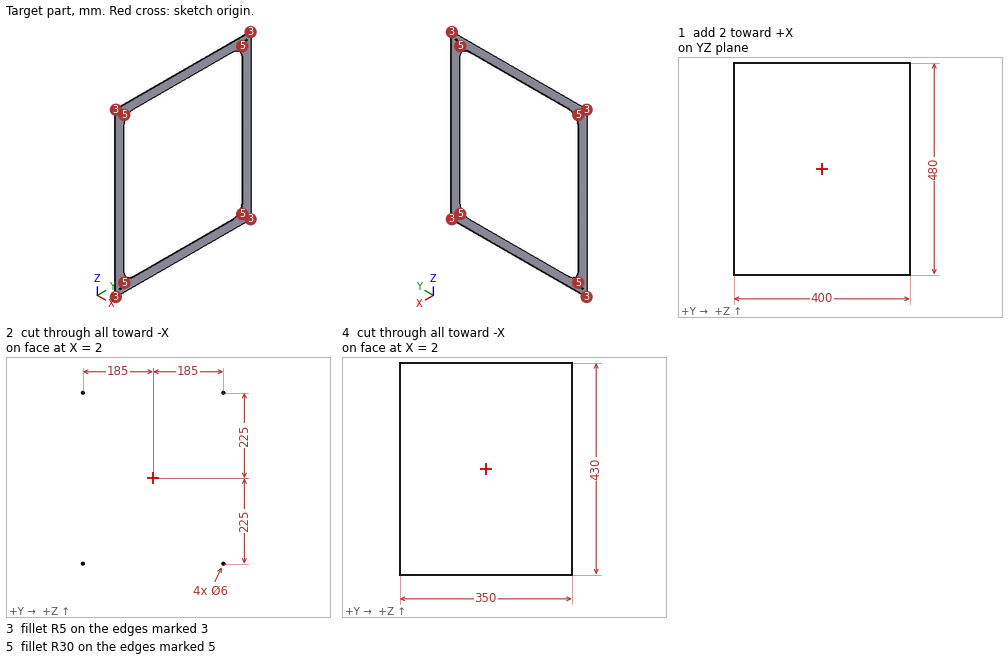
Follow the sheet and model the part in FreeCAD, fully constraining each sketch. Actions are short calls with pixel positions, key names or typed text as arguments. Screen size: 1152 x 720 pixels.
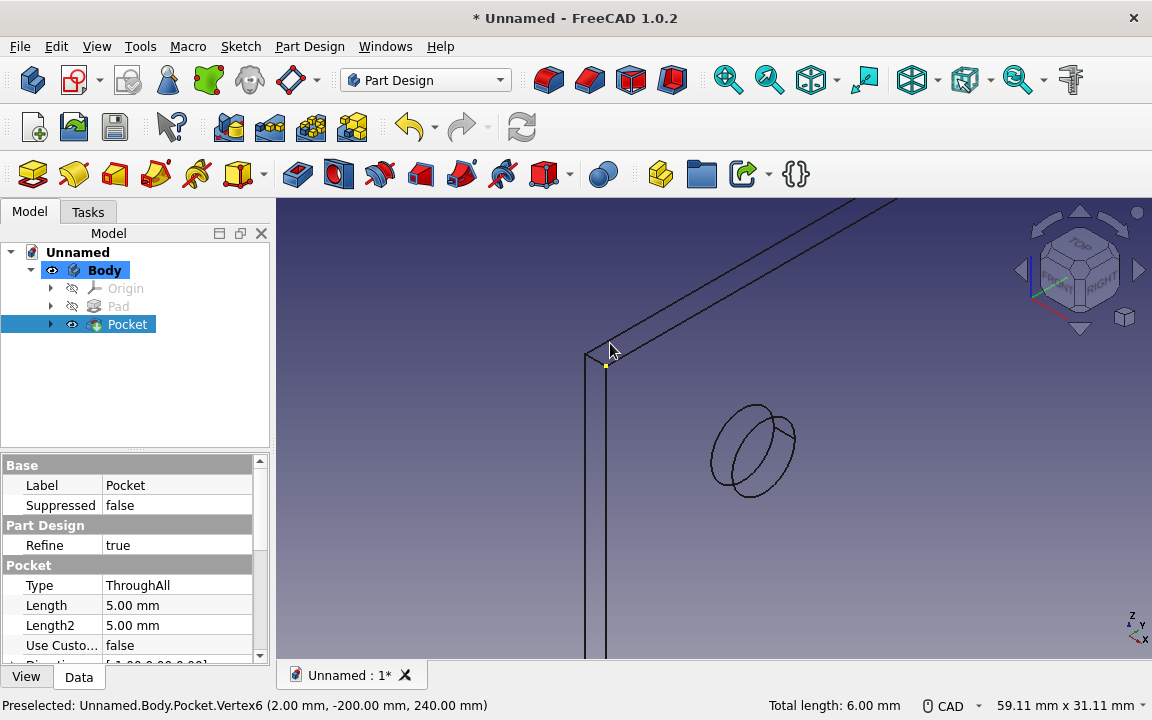
click(596, 359, ctrl)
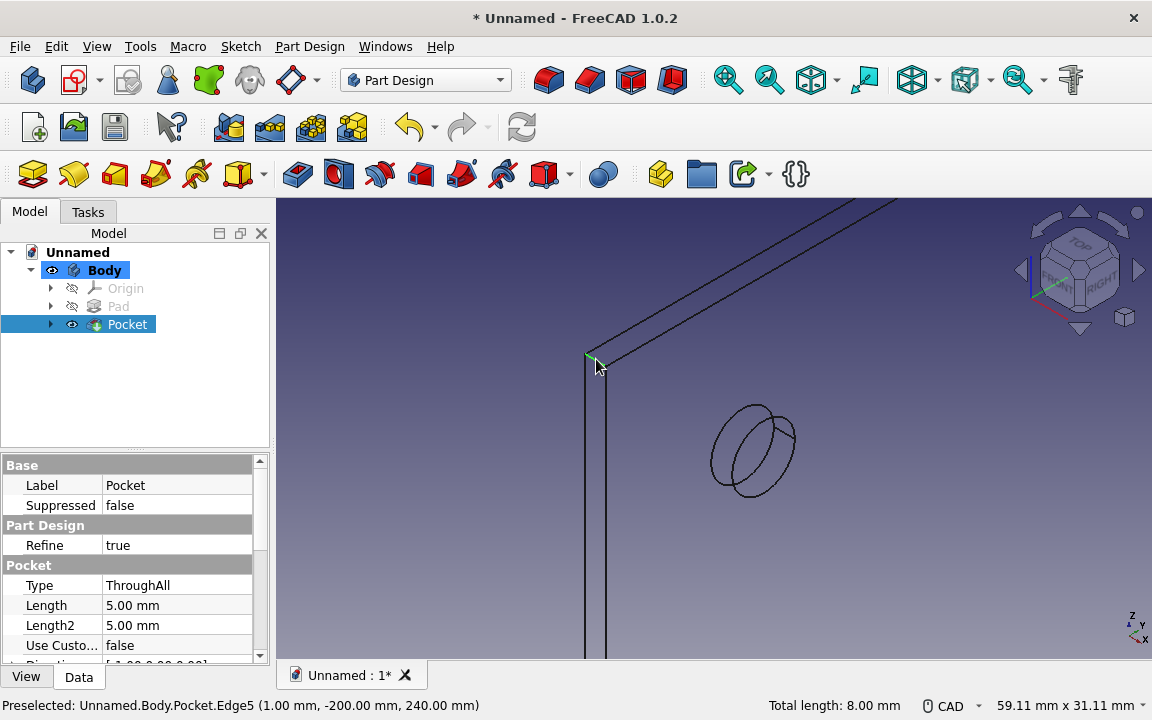
key(v)
key(1)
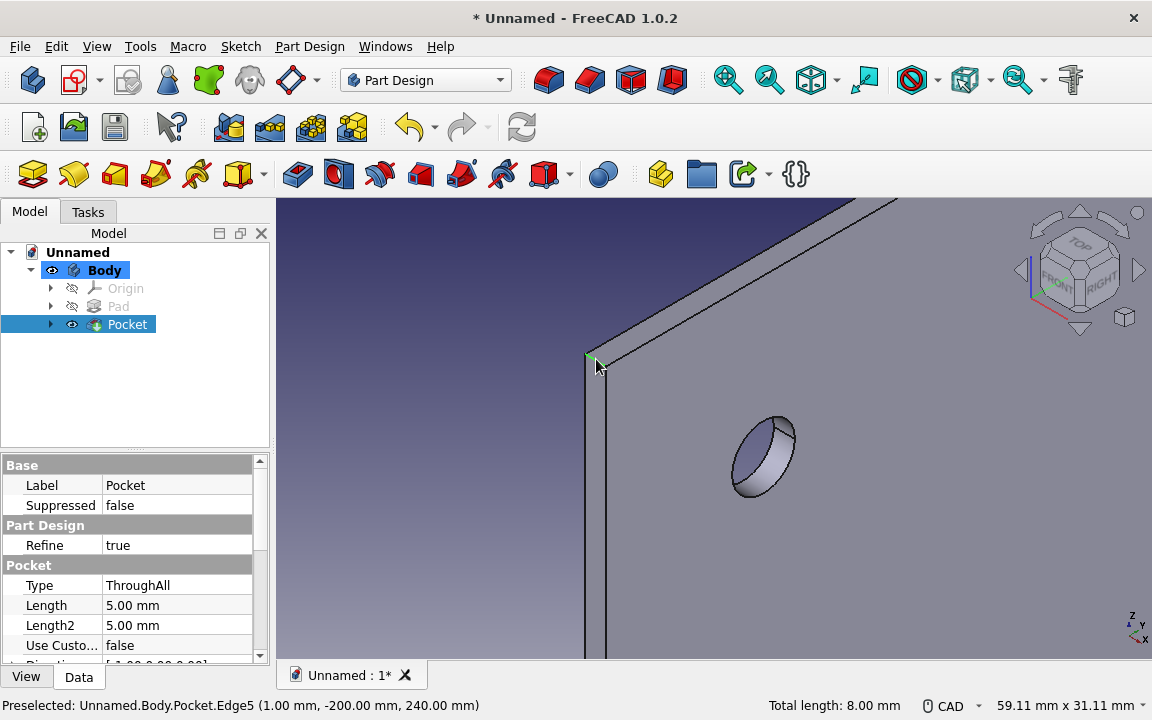
click(549, 80)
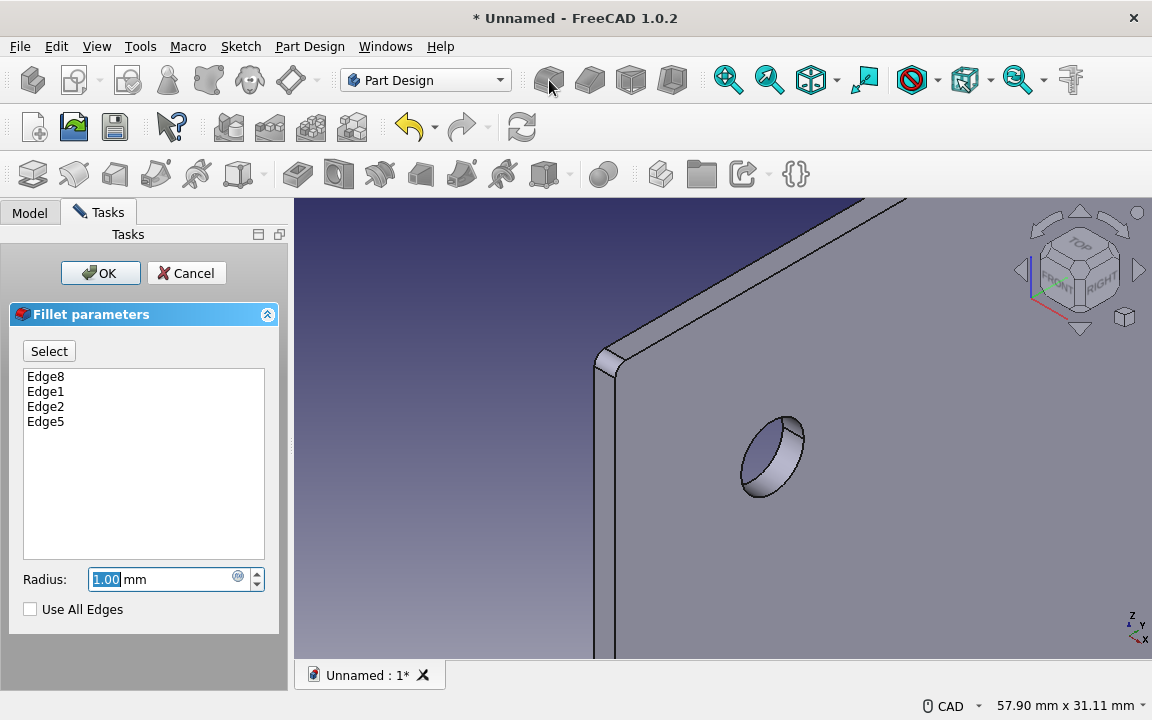
text(5)
key(Tab)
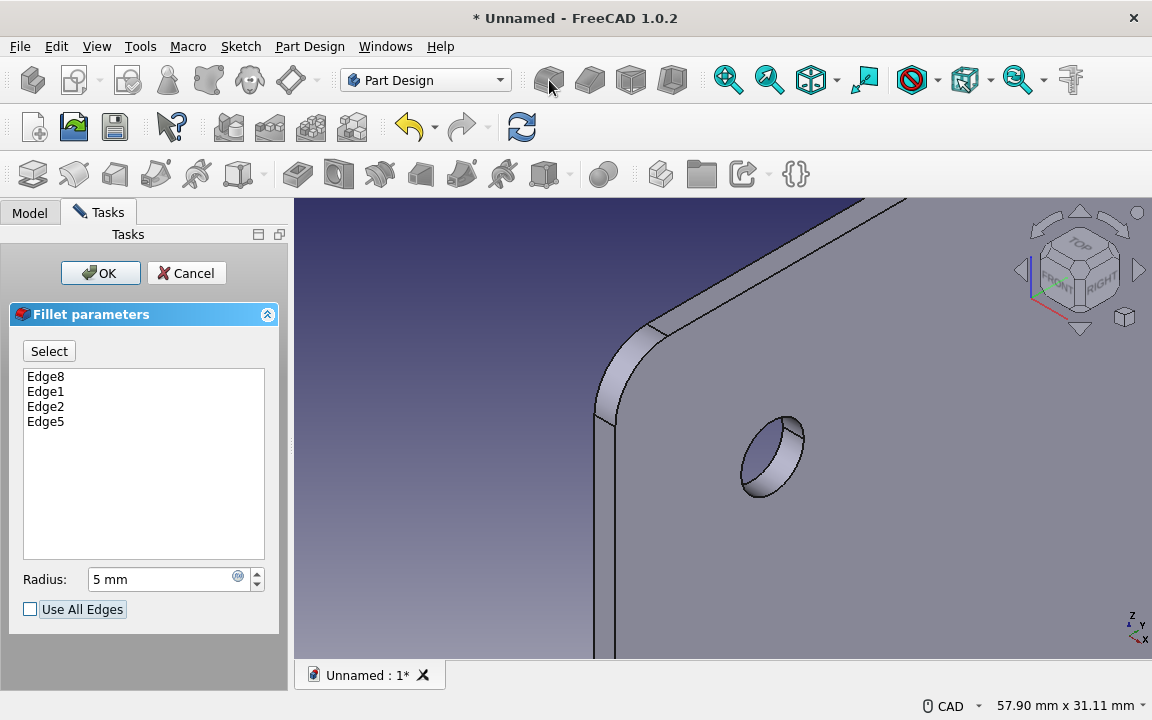
click(101, 273)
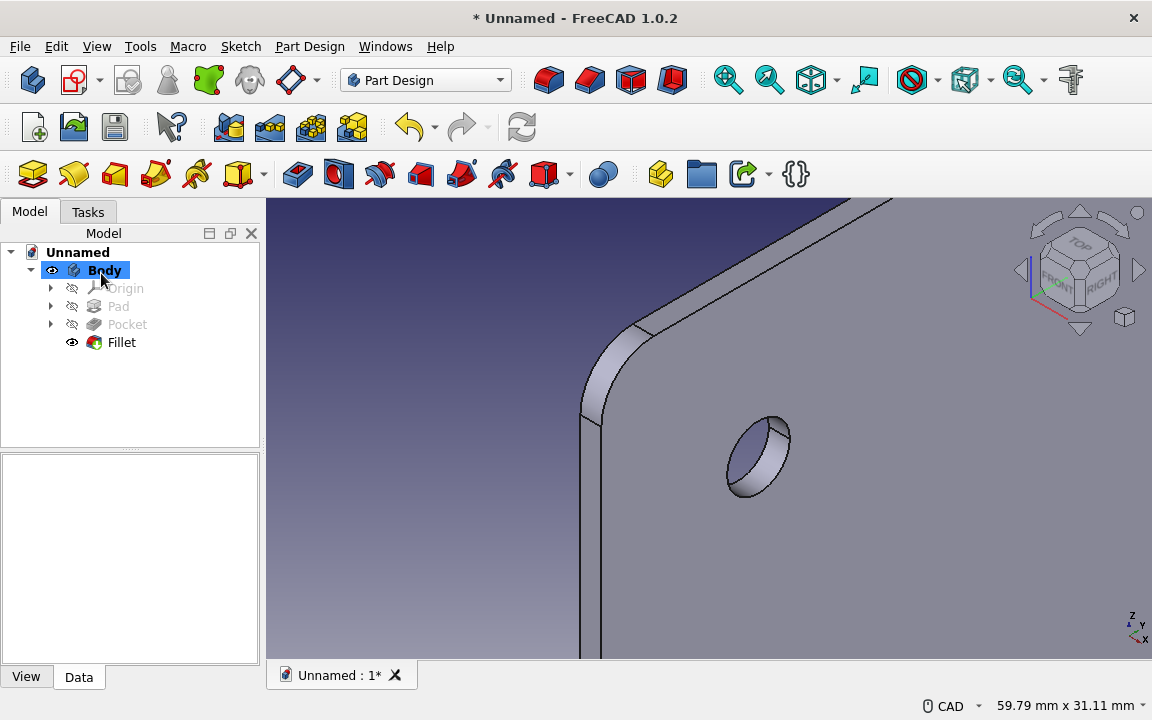
click(729, 80)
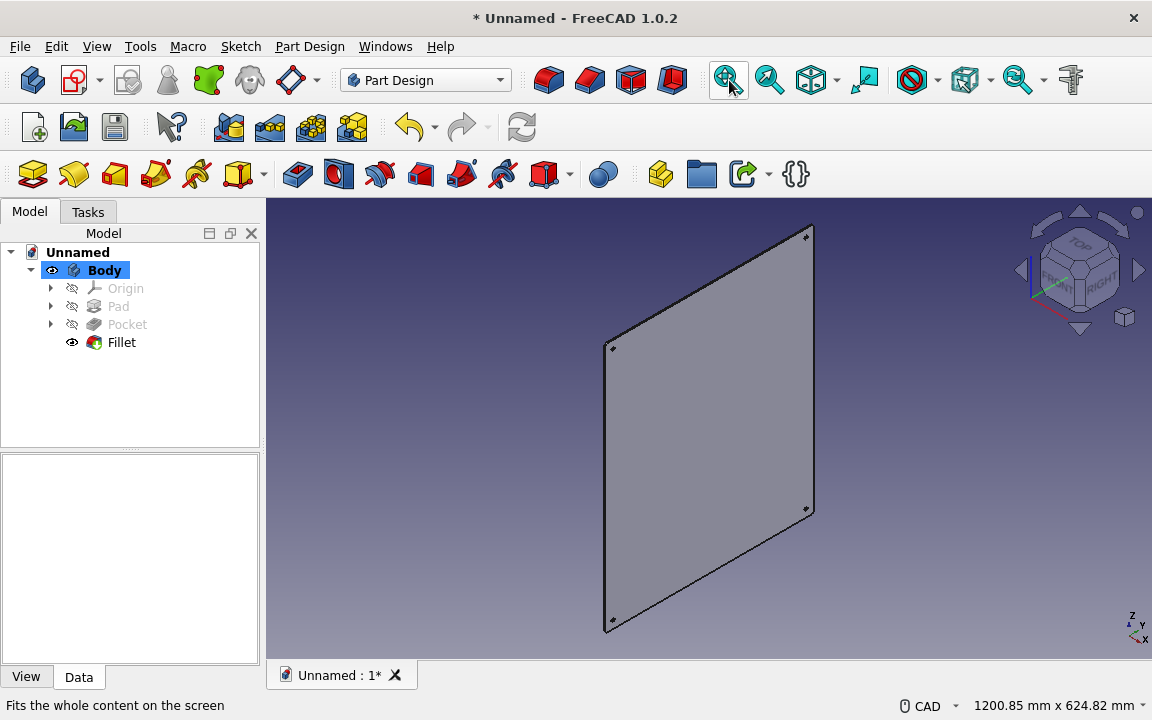
click(710, 428)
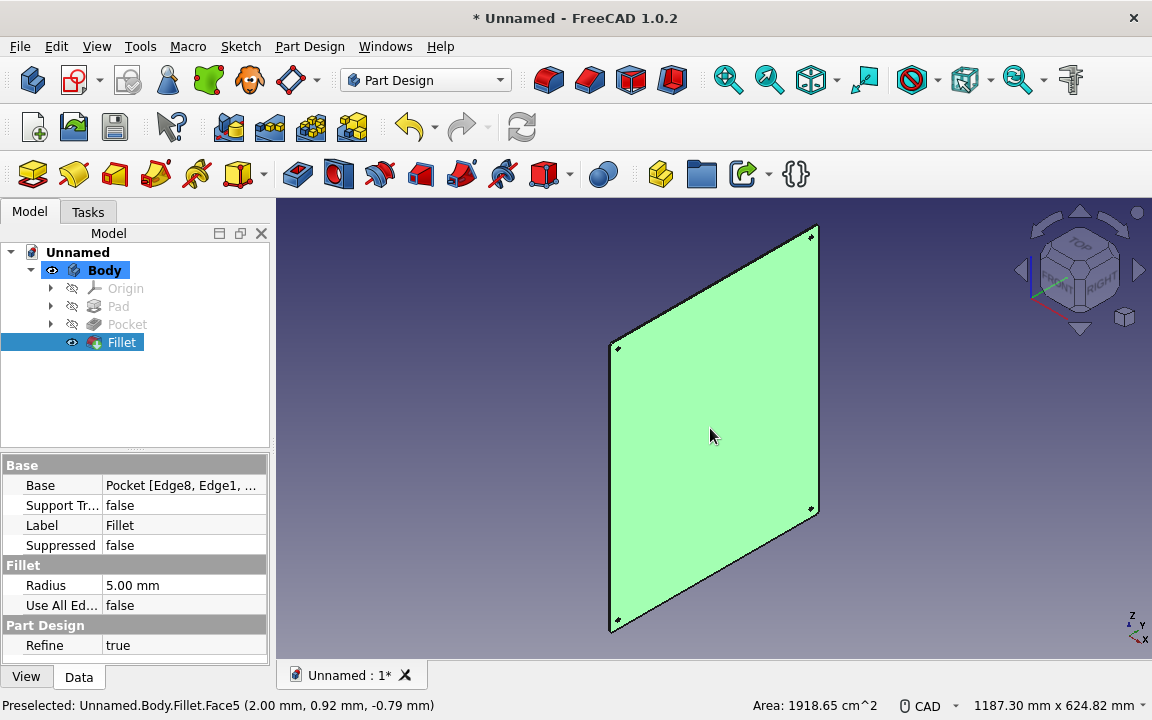
click(74, 80)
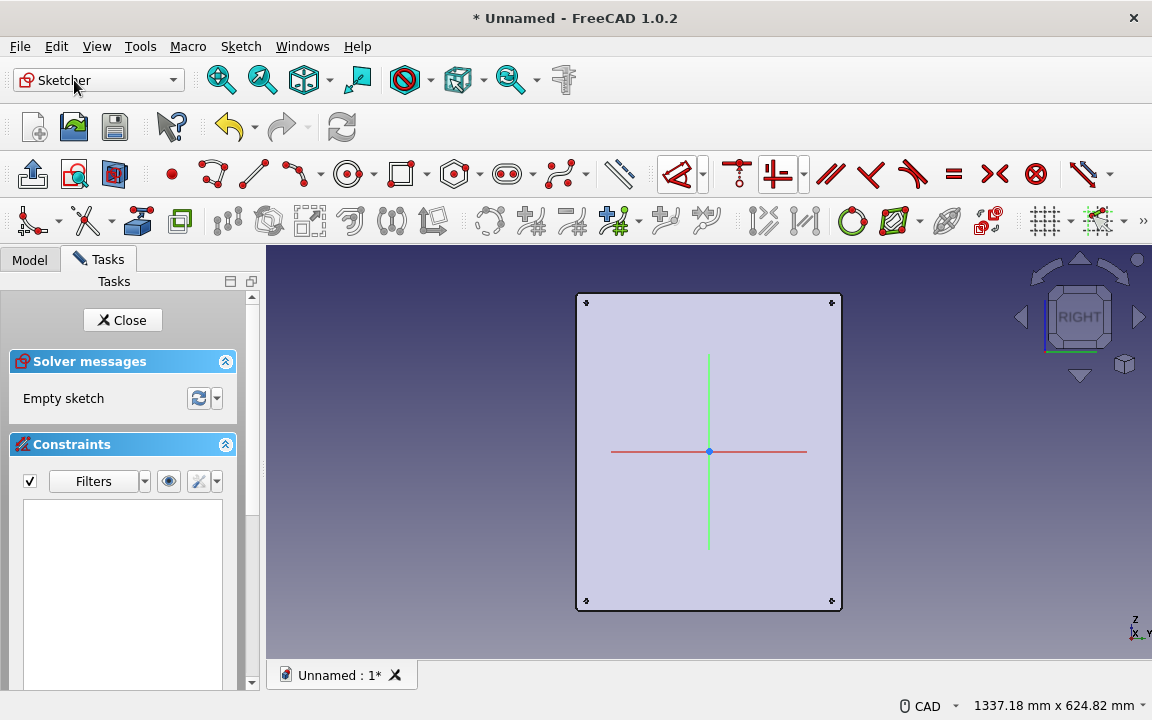
key(g)
key(v)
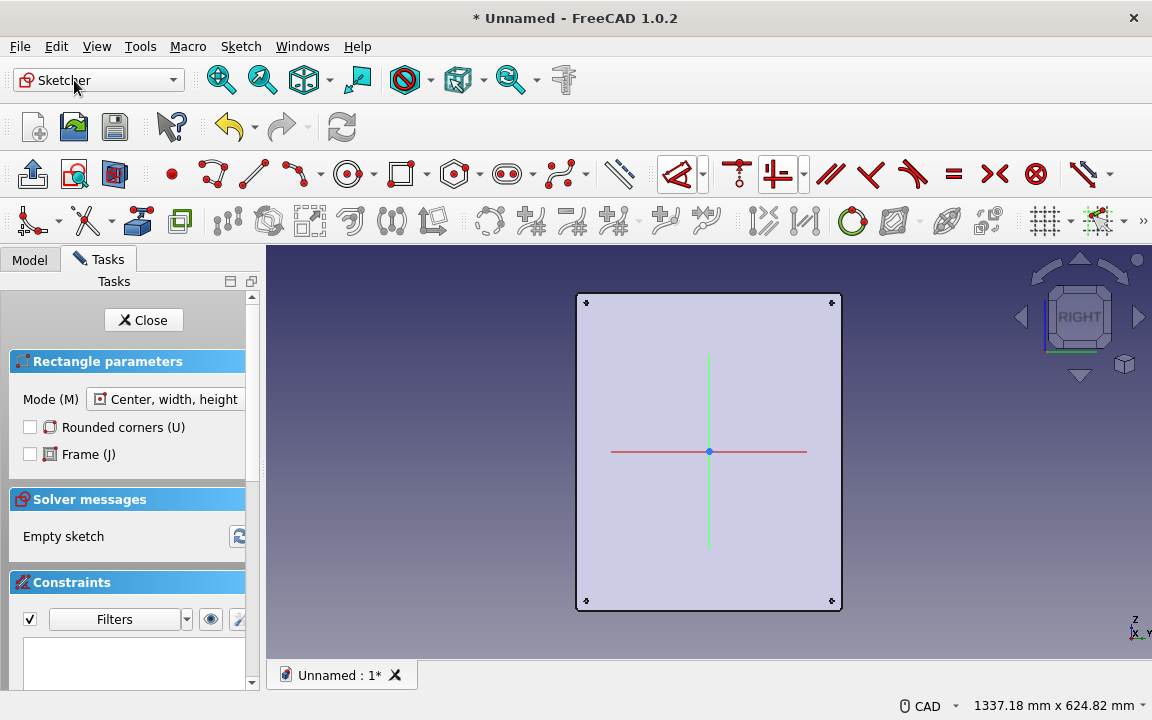
click(709, 452)
move(825, 310)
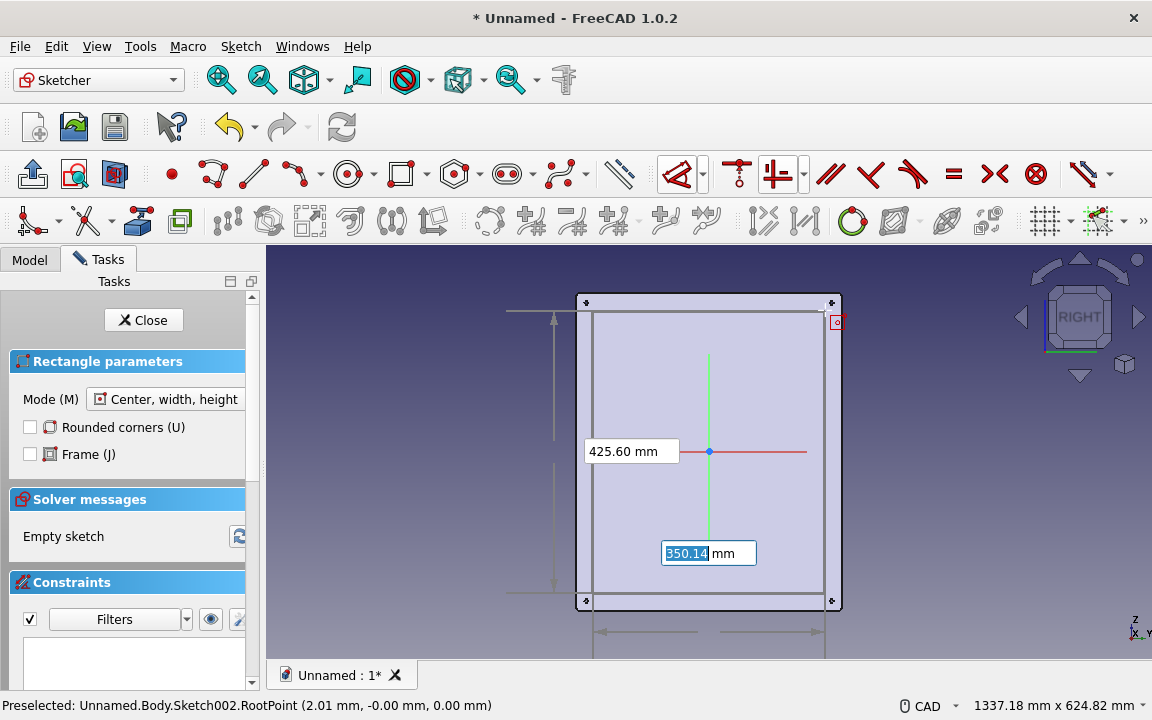
text(350)
key(Tab)
text(430)
key(Return)
key(Escape)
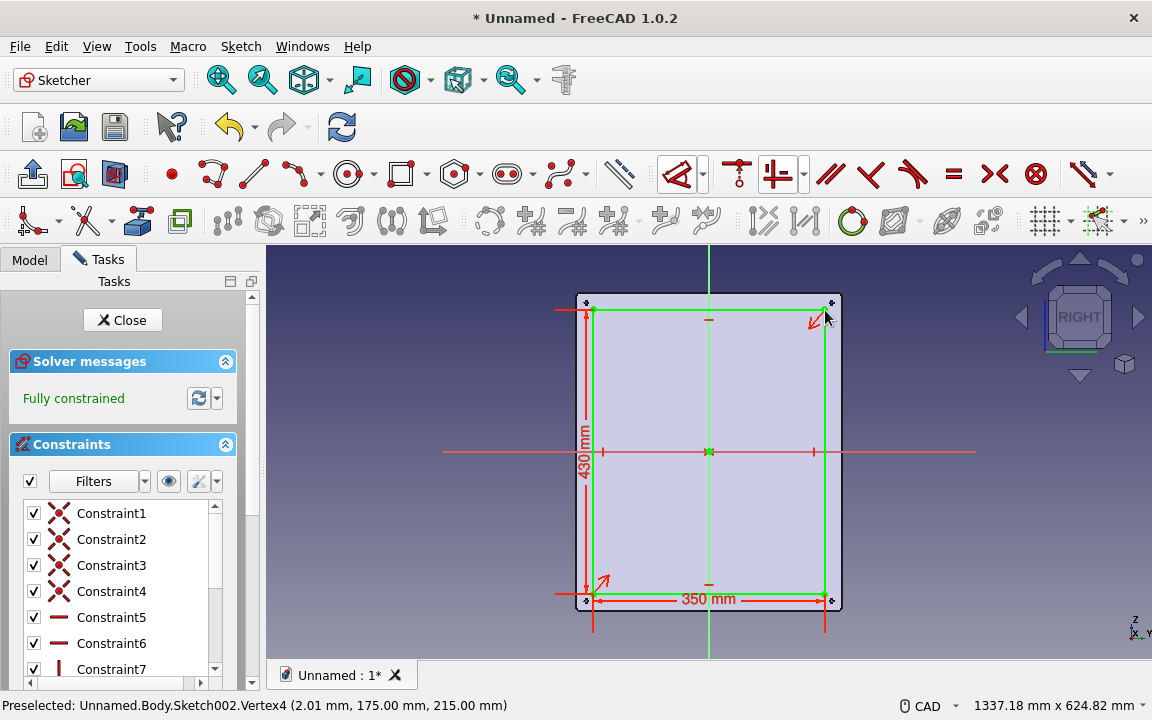
click(123, 320)